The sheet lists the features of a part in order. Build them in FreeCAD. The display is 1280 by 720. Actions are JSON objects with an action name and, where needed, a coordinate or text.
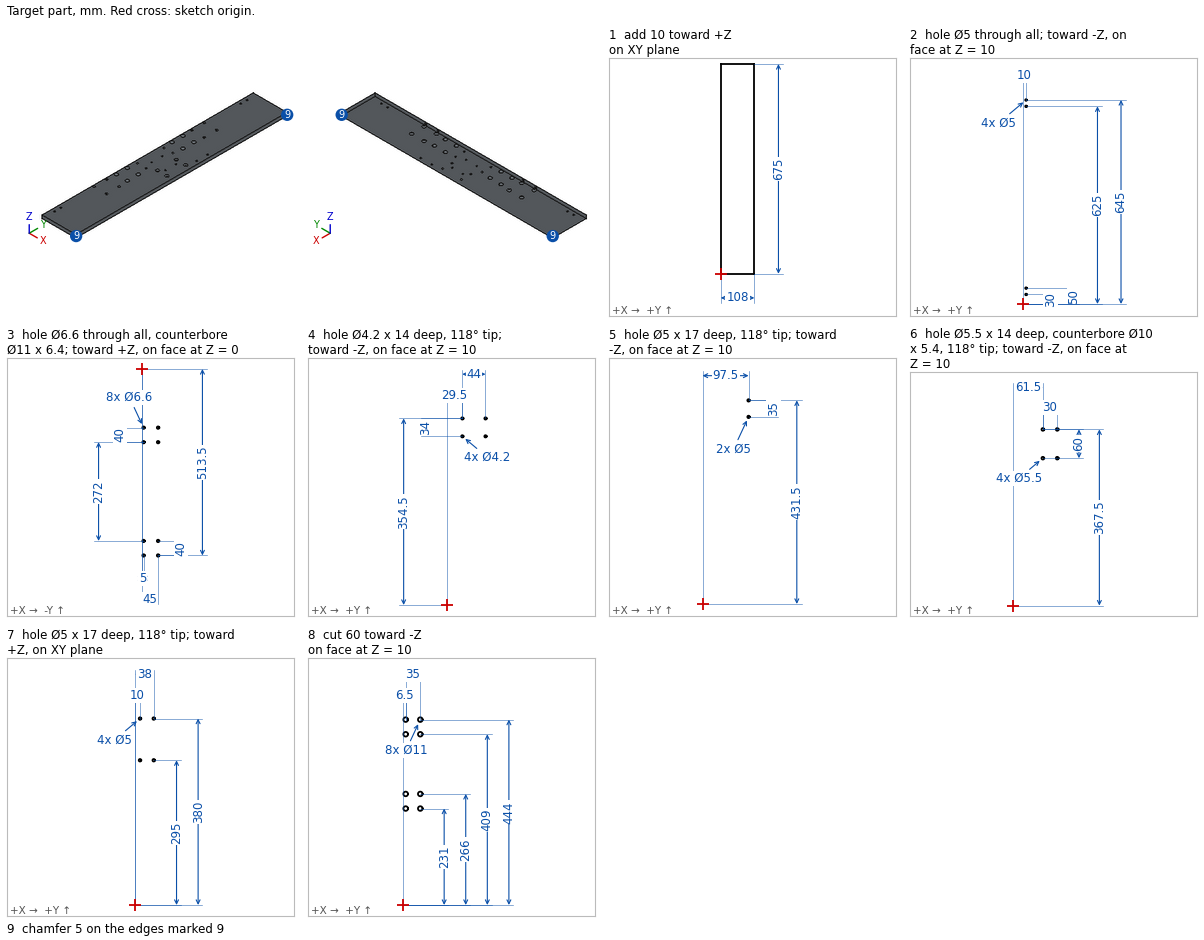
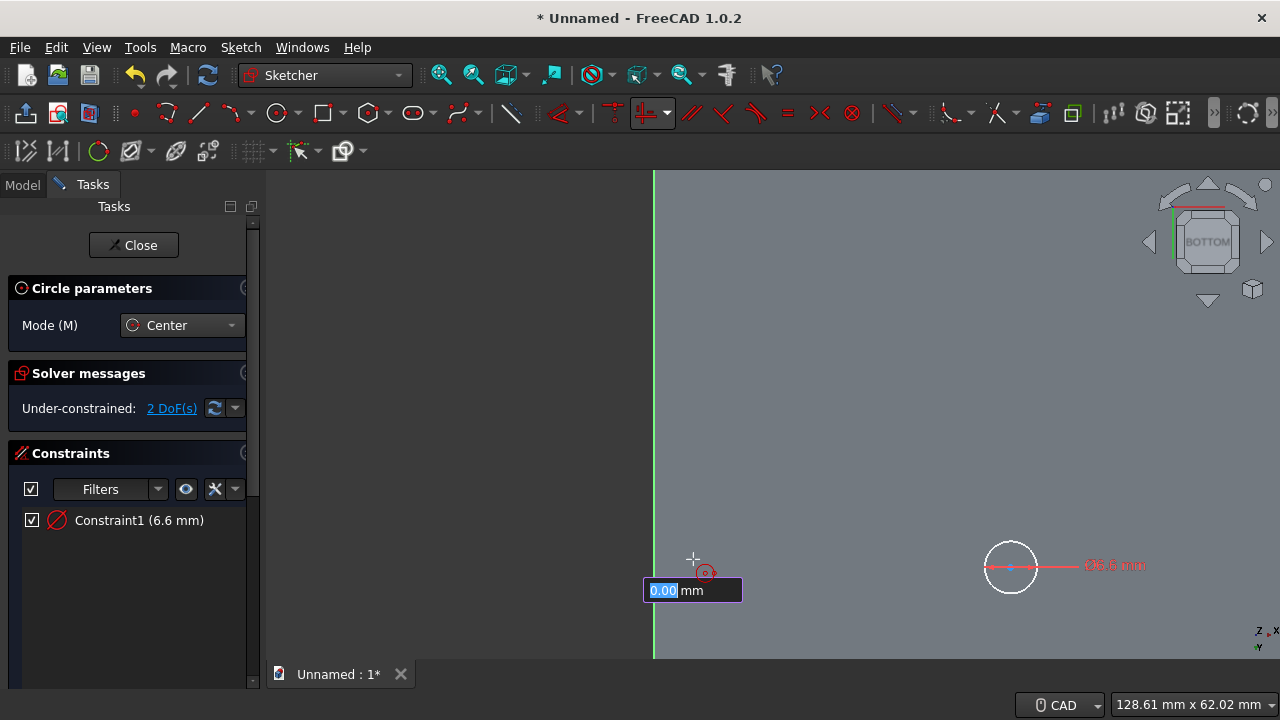
{"action": "scroll", "coordinate": [693, 564], "scroll_direction": "down", "scroll_amount": 13}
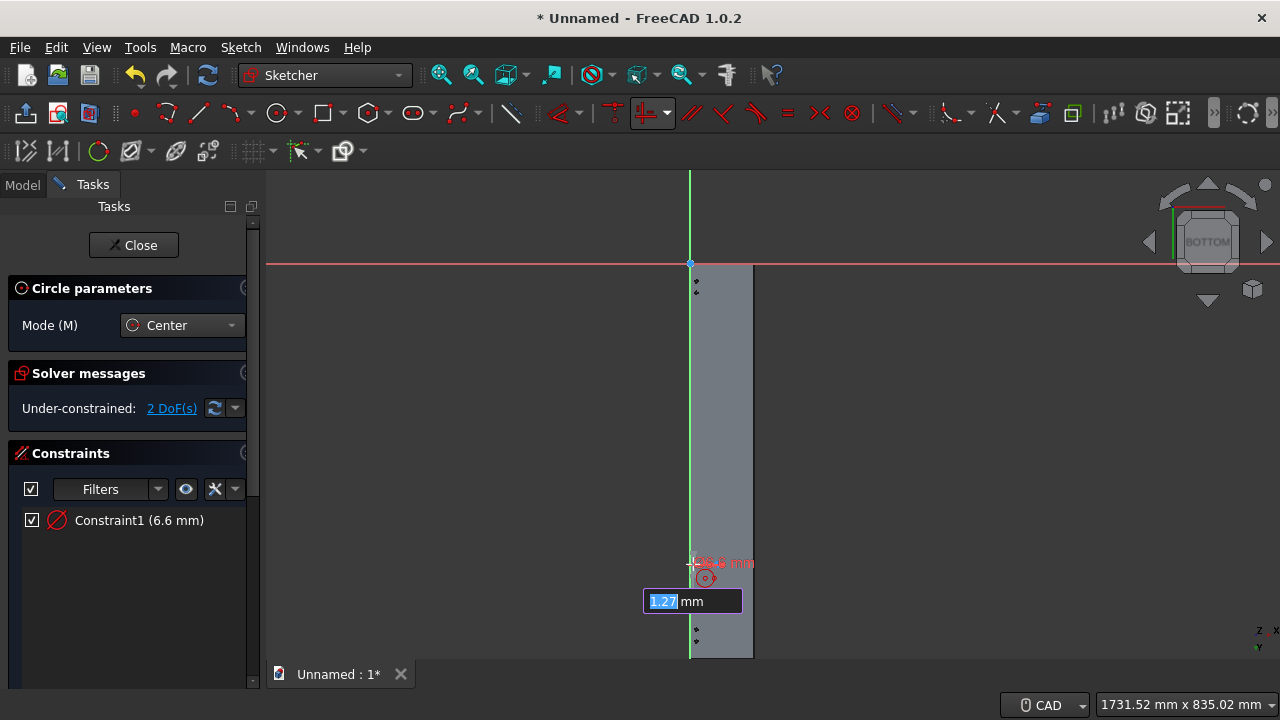
{"action": "scroll", "coordinate": [695, 563], "scroll_direction": "up", "scroll_amount": 7}
{"action": "mouse_move", "coordinate": [693, 561]}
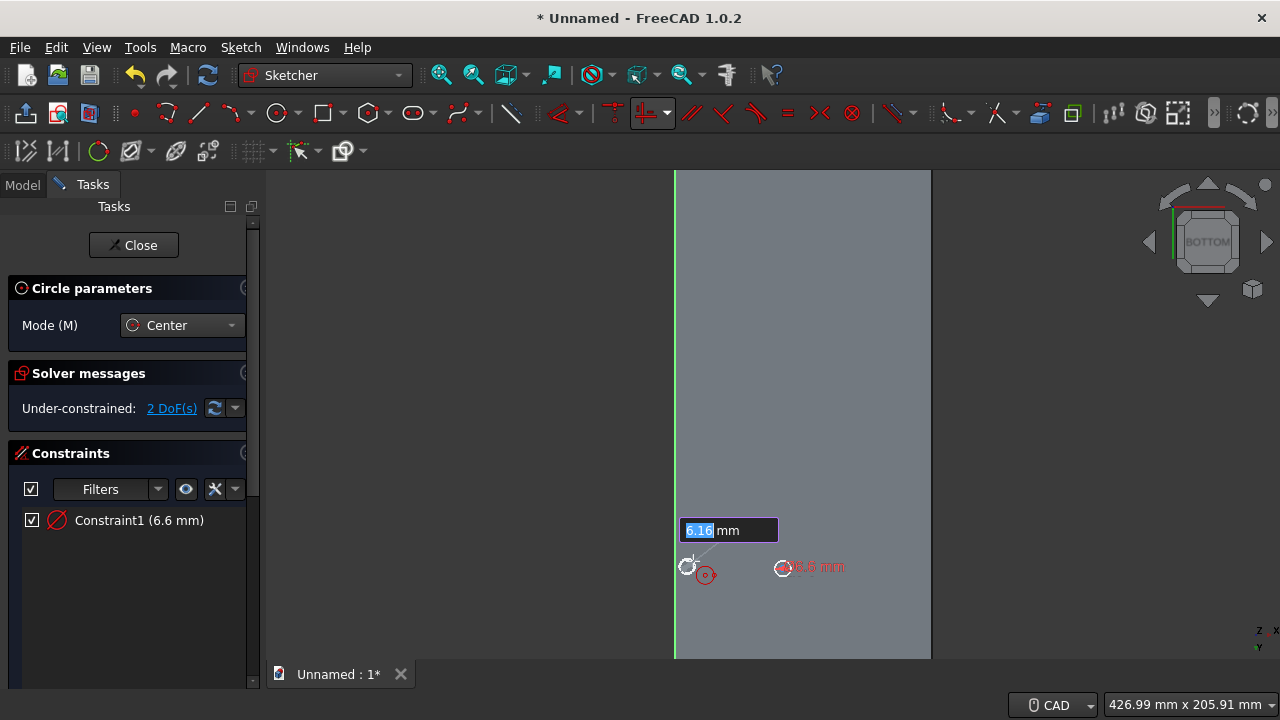
{"action": "type", "text": "6.6"}
{"action": "key", "text": "Return"}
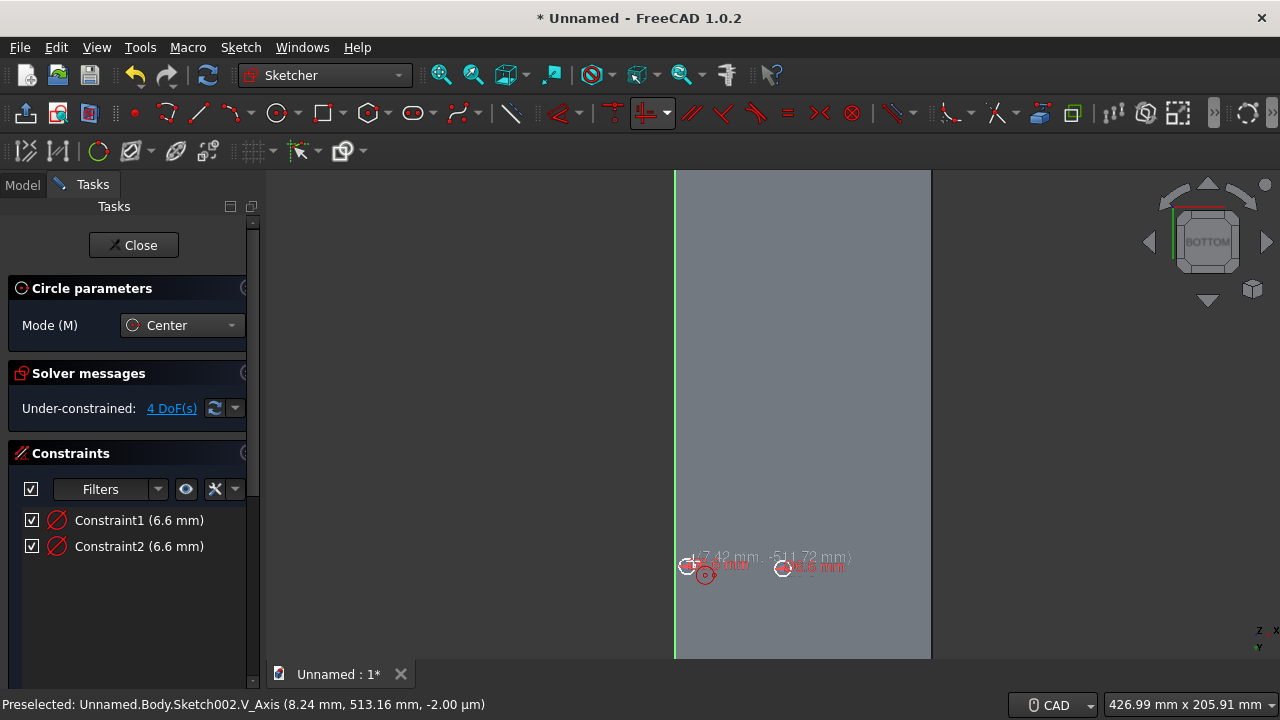
{"action": "scroll", "coordinate": [782, 471], "scroll_direction": "up", "scroll_amount": 6}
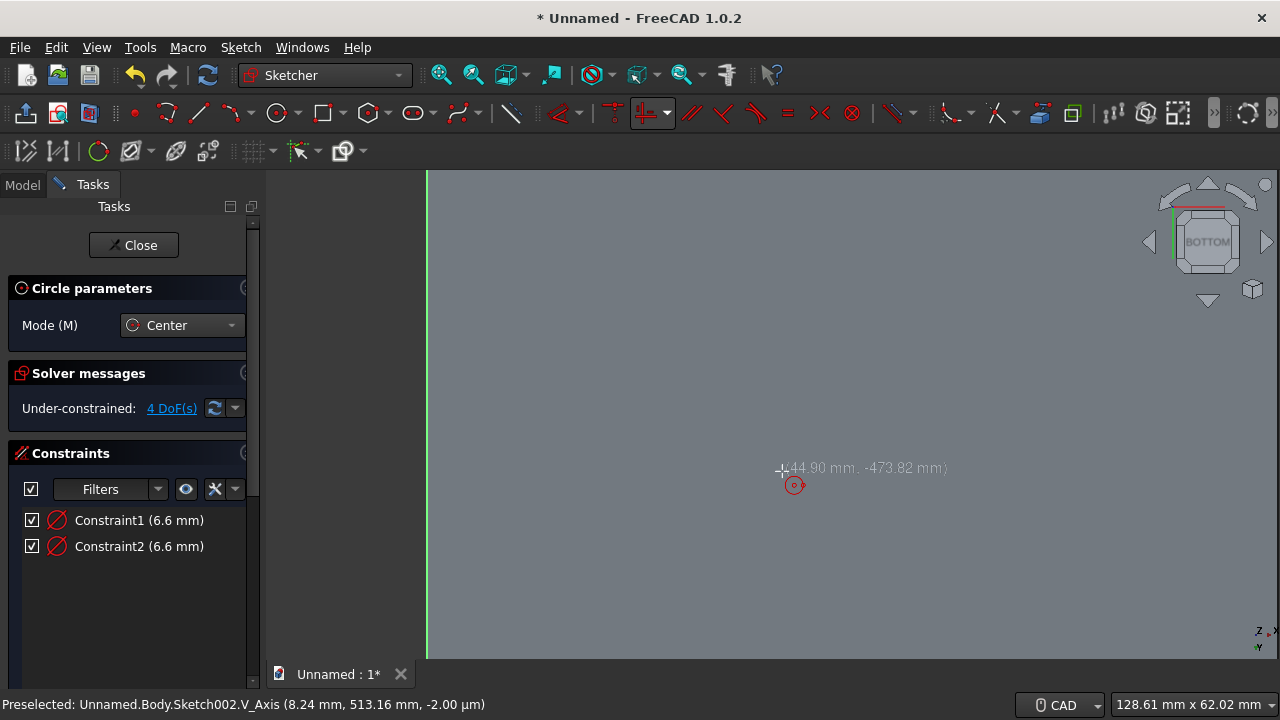
{"action": "scroll", "coordinate": [712, 546], "scroll_direction": "down", "scroll_amount": 13}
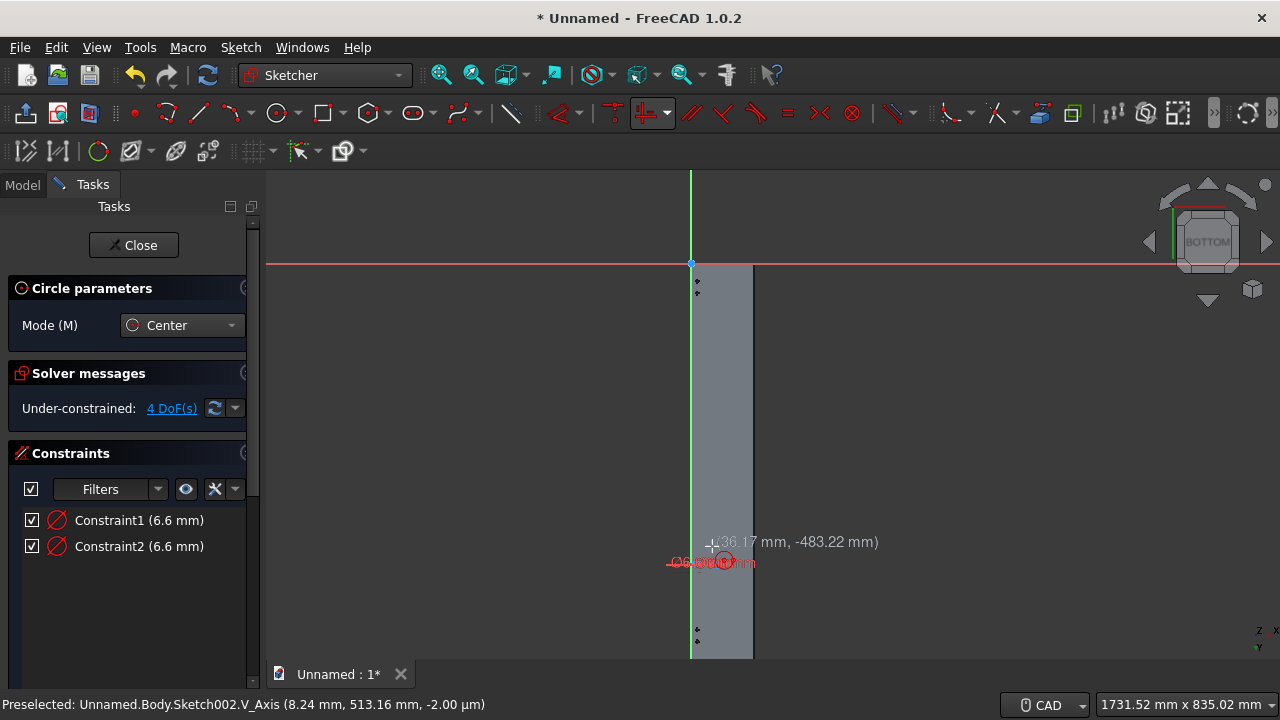
{"action": "left_click", "coordinate": [718, 541]}
{"action": "mouse_move", "coordinate": [719, 540]}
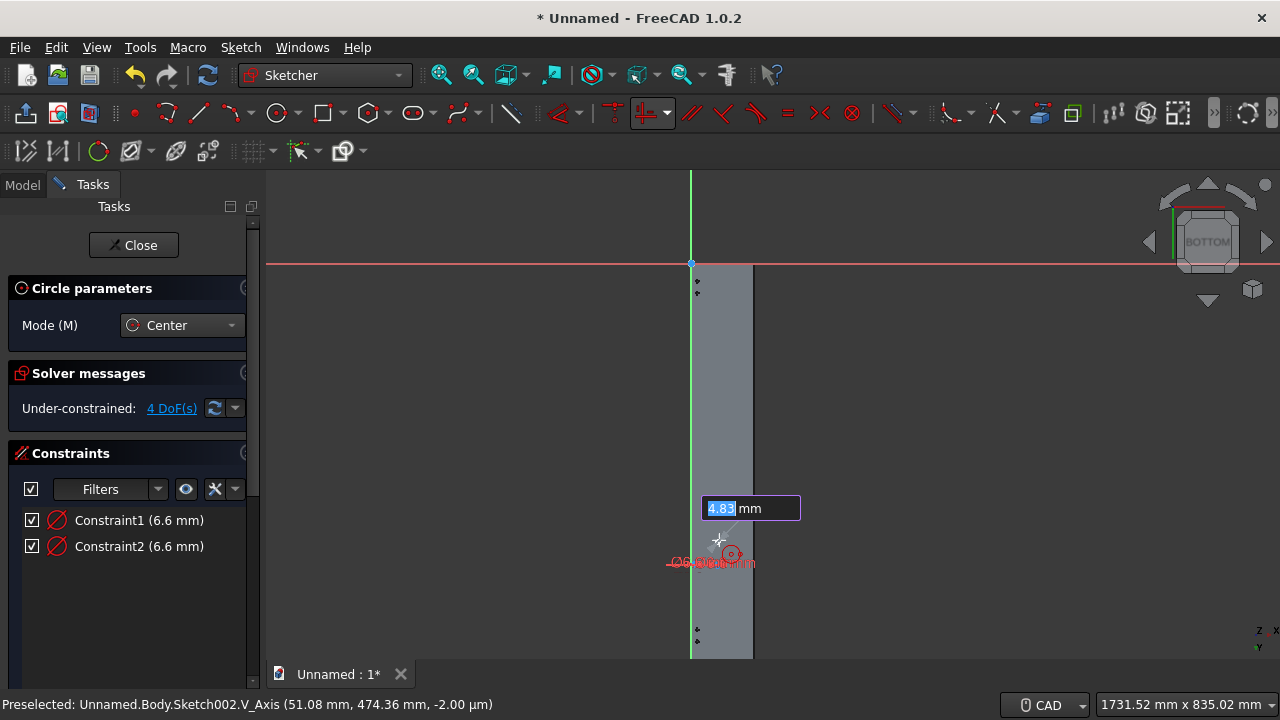
{"action": "type", "text": "6.6"}
{"action": "key", "text": "Return"}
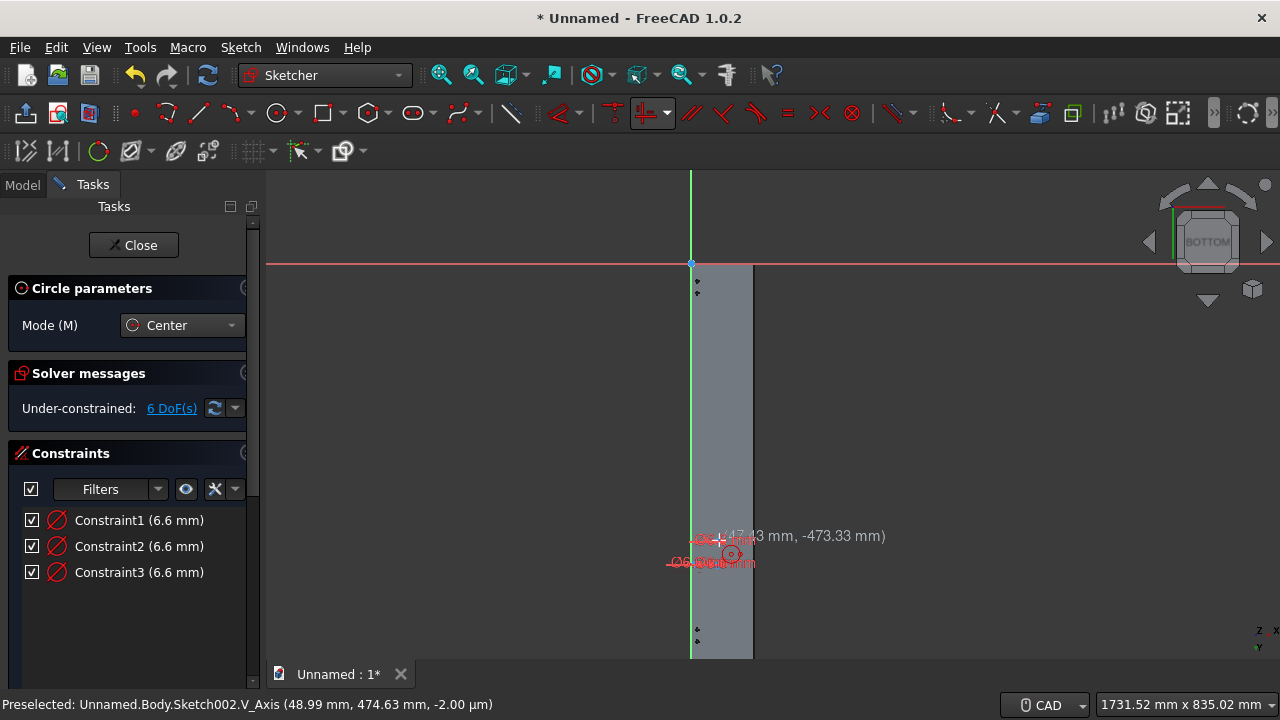
{"action": "scroll", "coordinate": [694, 541], "scroll_direction": "up", "scroll_amount": 13}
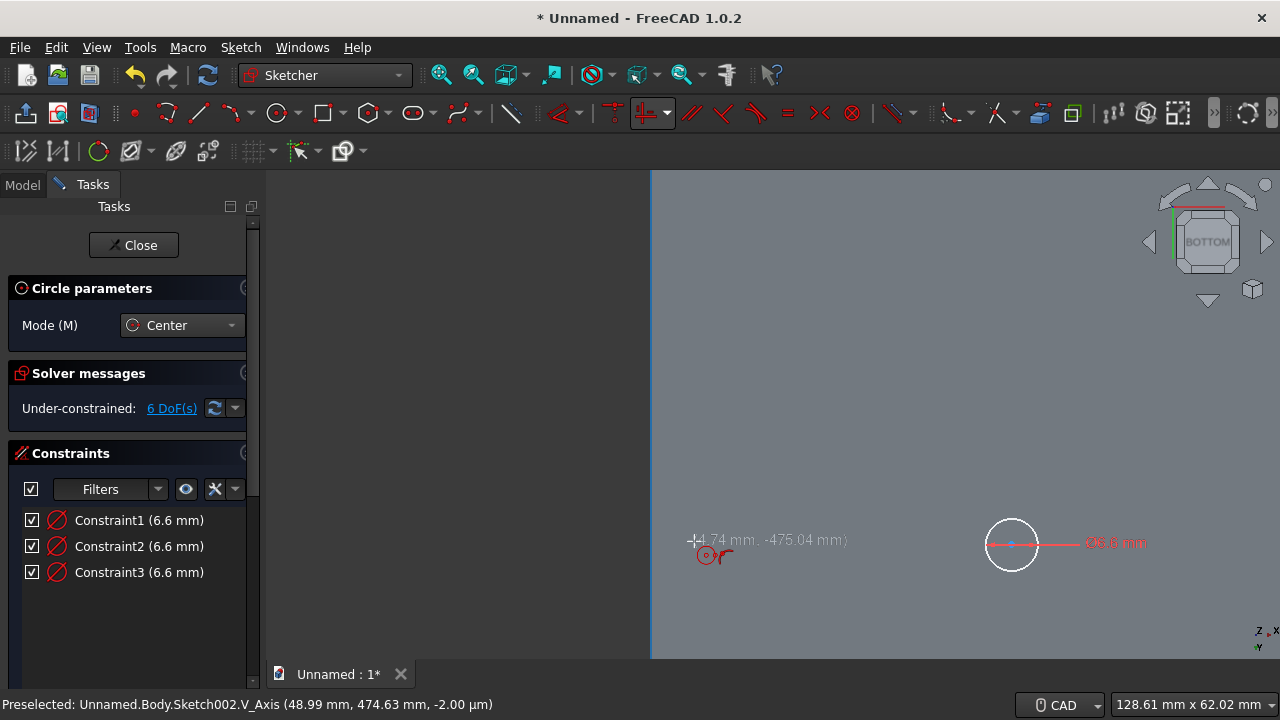
{"action": "left_click", "coordinate": [691, 533]}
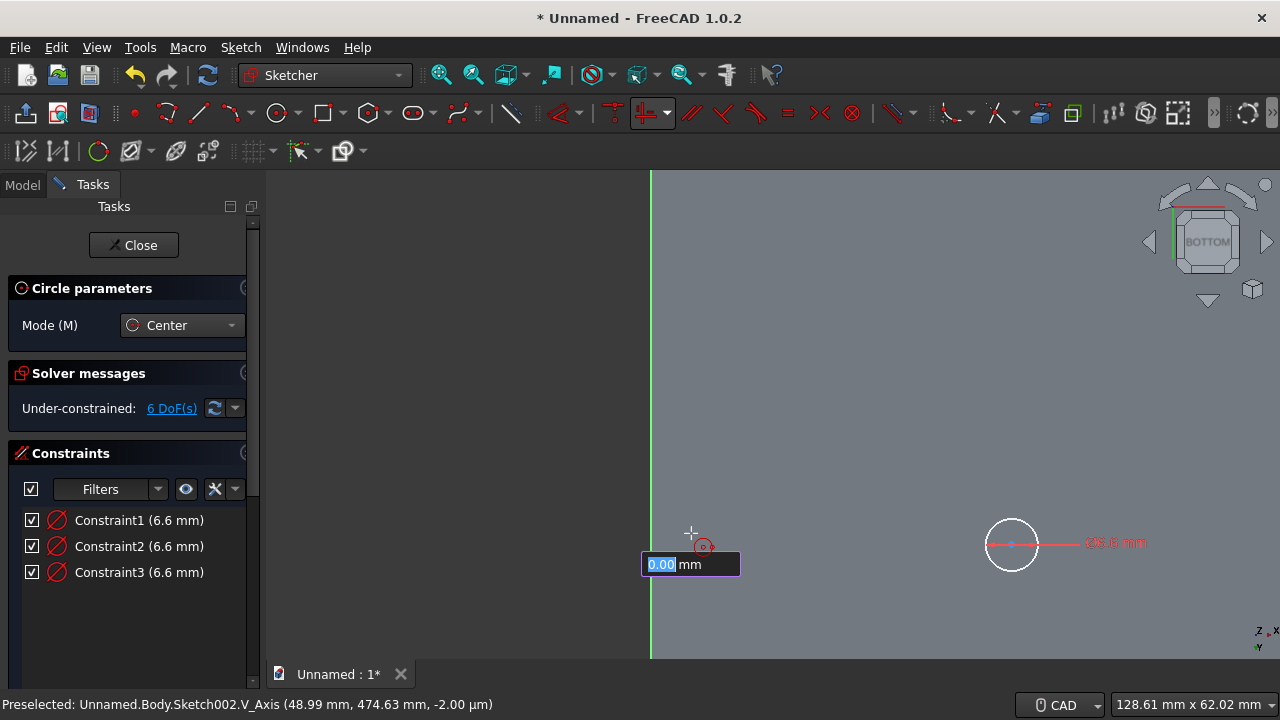
{"action": "scroll", "coordinate": [693, 541], "scroll_direction": "down", "scroll_amount": 13}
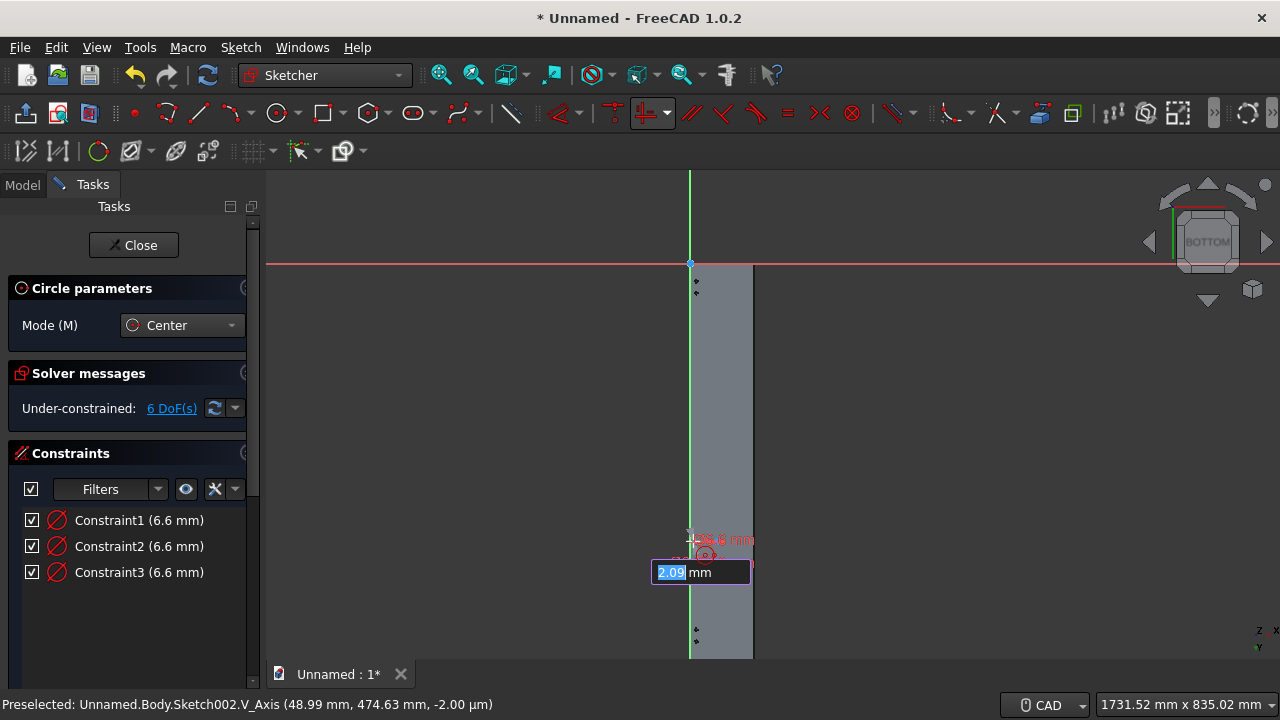
{"action": "scroll", "coordinate": [695, 540], "scroll_direction": "up", "scroll_amount": 7}
{"action": "mouse_move", "coordinate": [692, 537]}